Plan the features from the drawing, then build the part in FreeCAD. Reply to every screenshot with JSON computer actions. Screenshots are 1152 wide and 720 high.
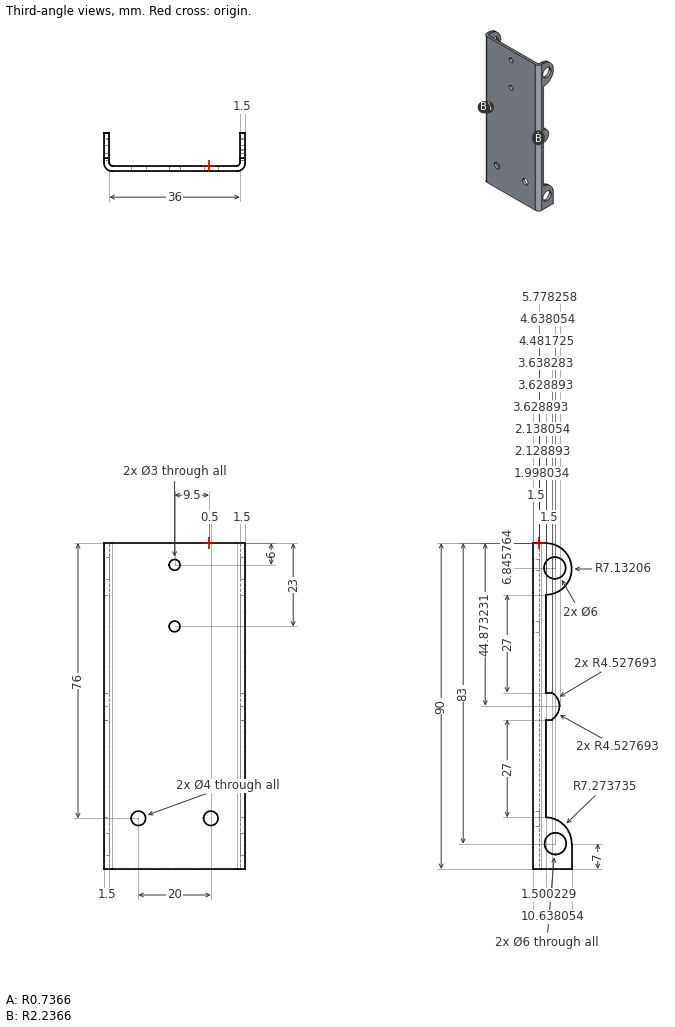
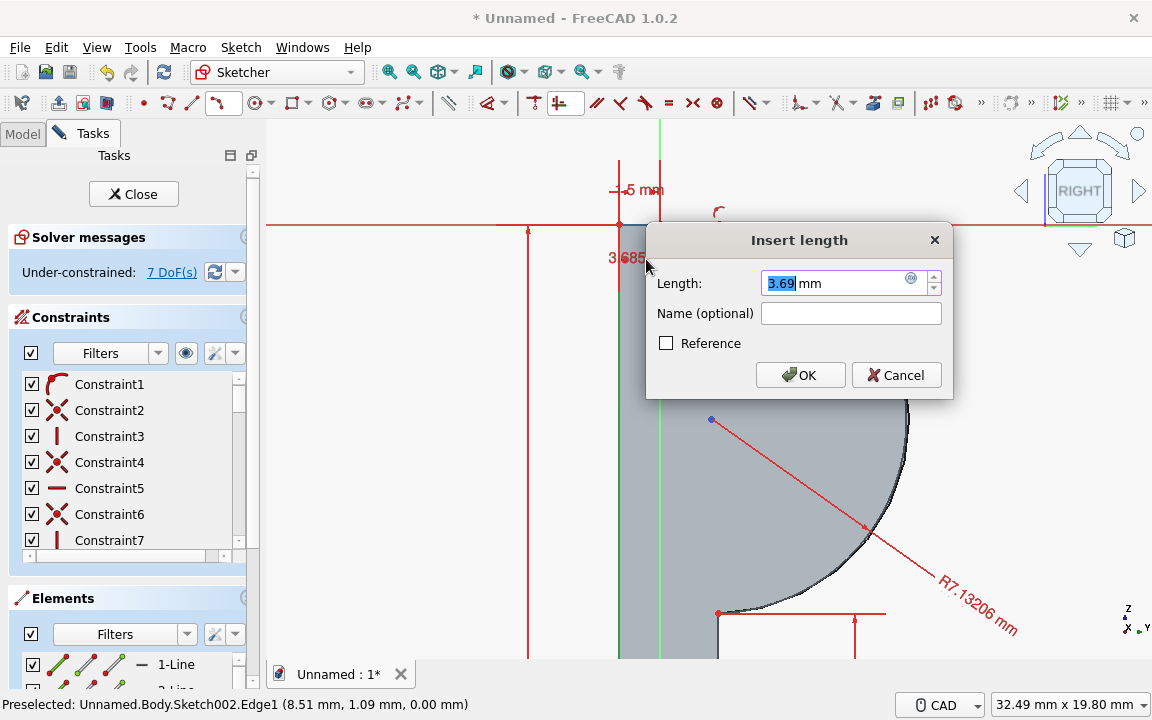
{"action": "type", "text": "3.628893"}
{"action": "key", "text": "Return"}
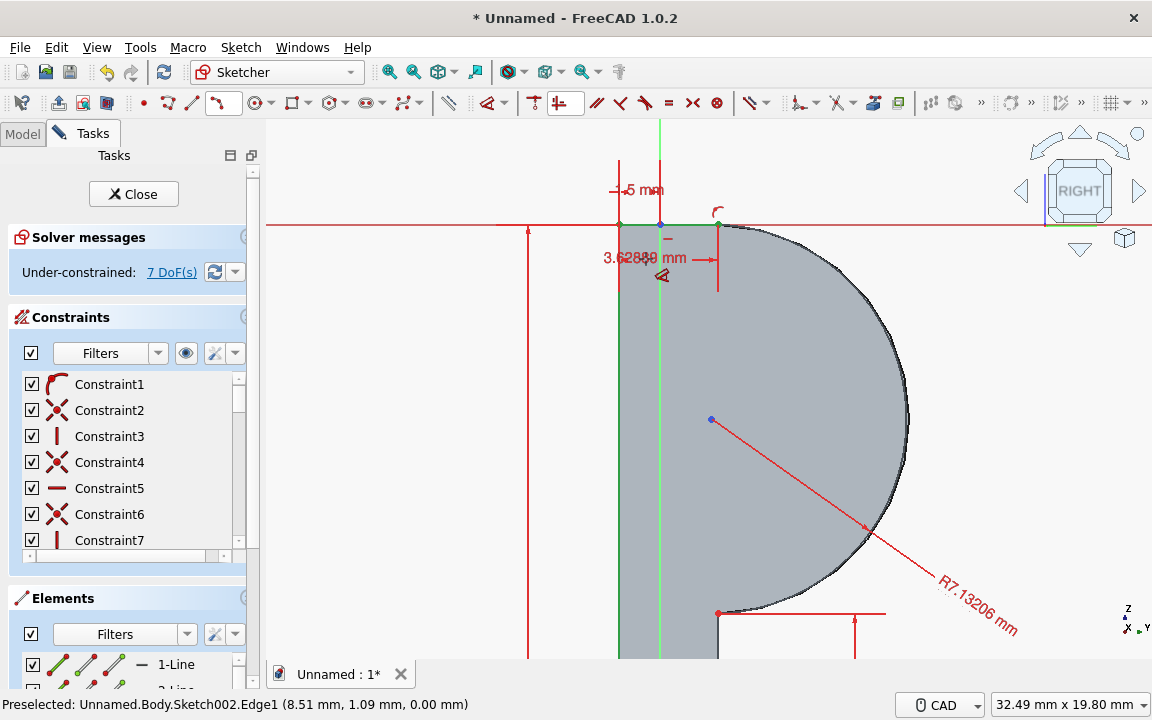
{"action": "scroll", "coordinate": [621, 223], "scroll_direction": "down", "scroll_amount": 10}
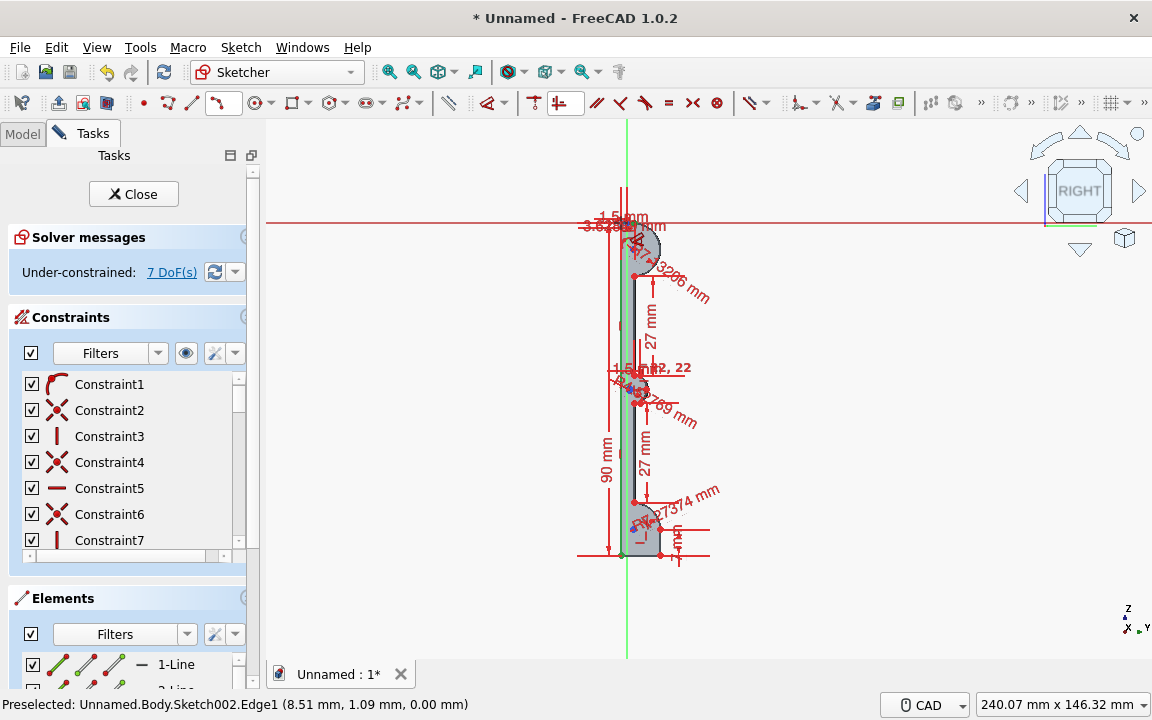
{"action": "scroll", "coordinate": [636, 403], "scroll_direction": "up", "scroll_amount": 11}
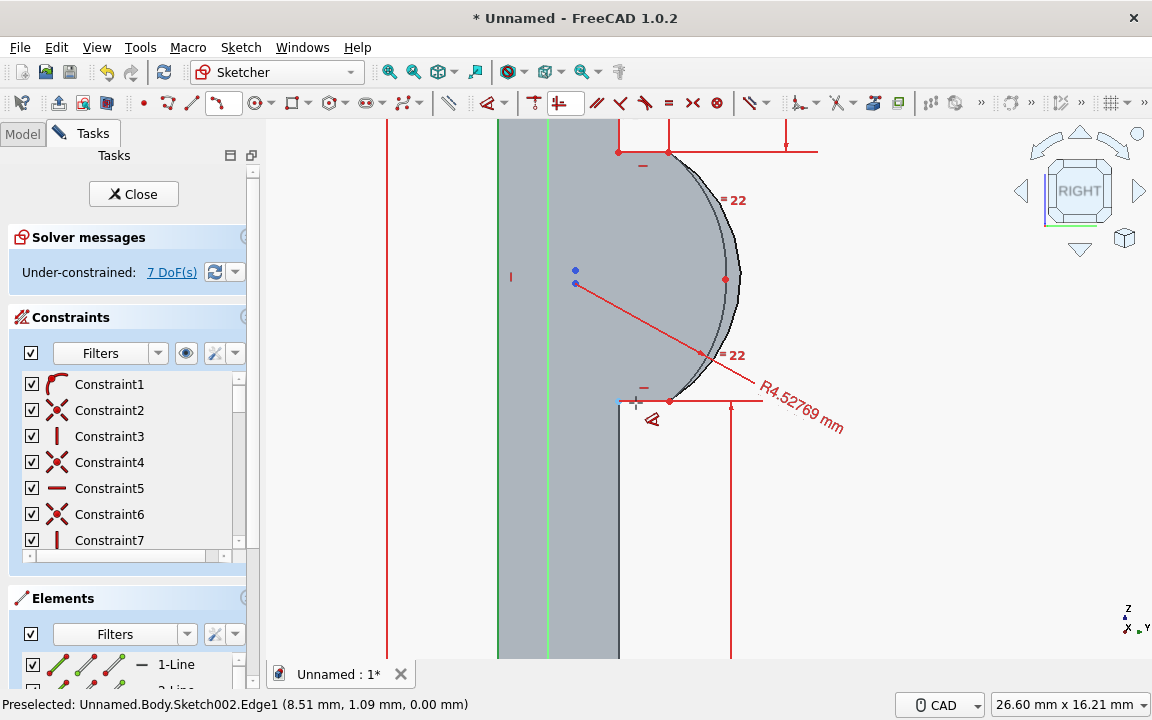
{"action": "left_click", "coordinate": [634, 401]}
{"action": "left_click", "coordinate": [644, 435]}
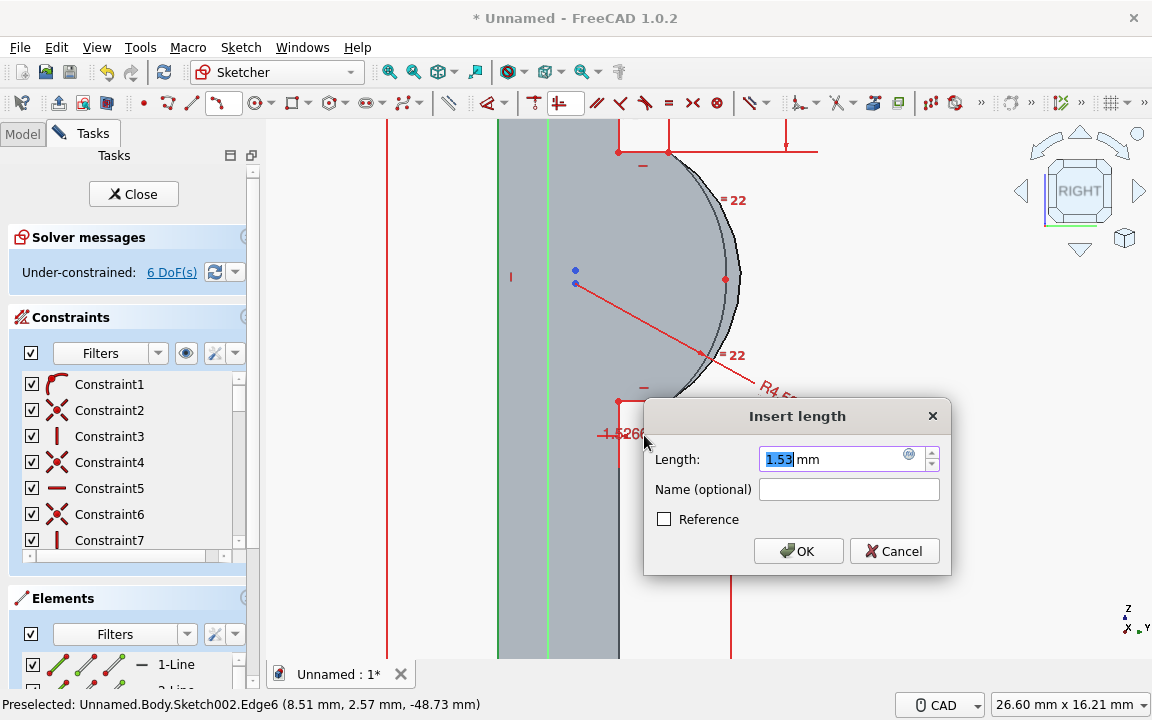
{"action": "type", "text": "1.500229"}
{"action": "key", "text": "Return"}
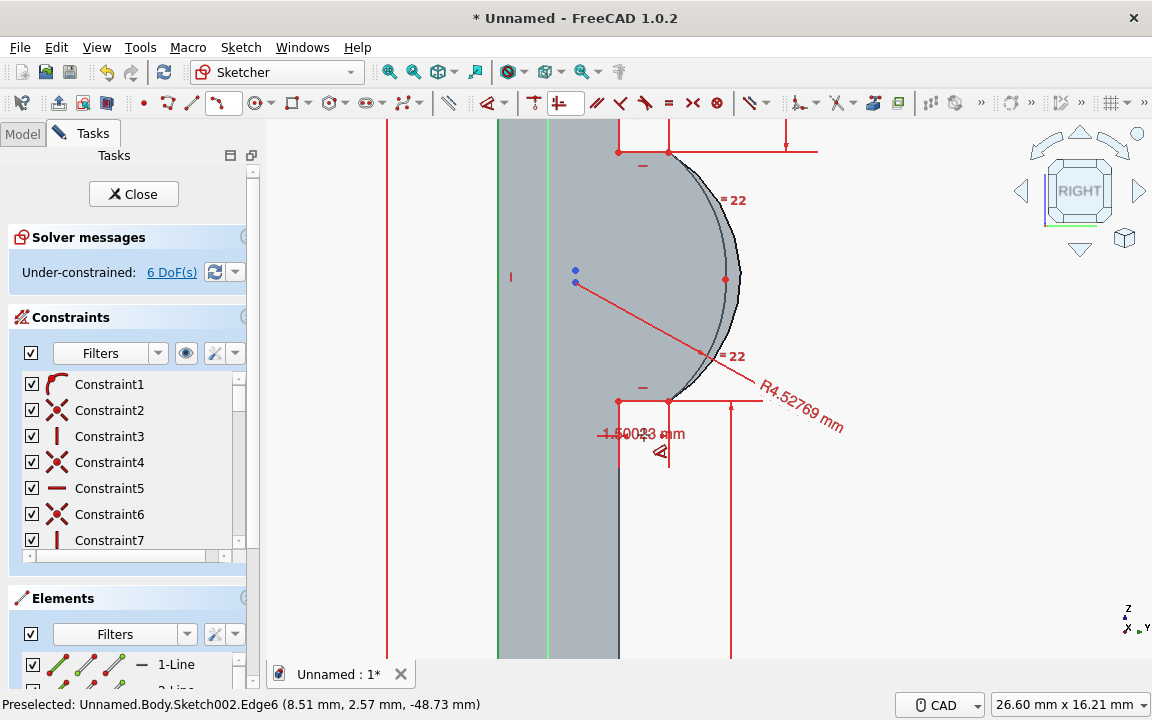
{"action": "scroll", "coordinate": [636, 403], "scroll_direction": "down", "scroll_amount": 11}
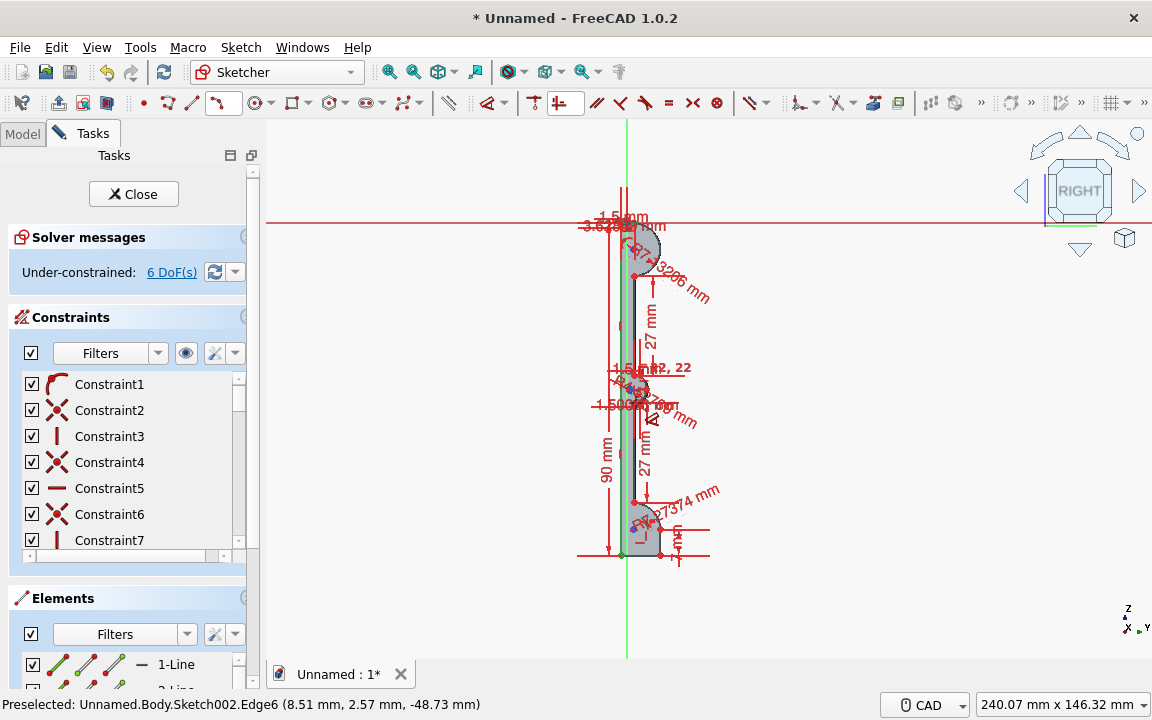
{"action": "scroll", "coordinate": [633, 556], "scroll_direction": "up", "scroll_amount": 4}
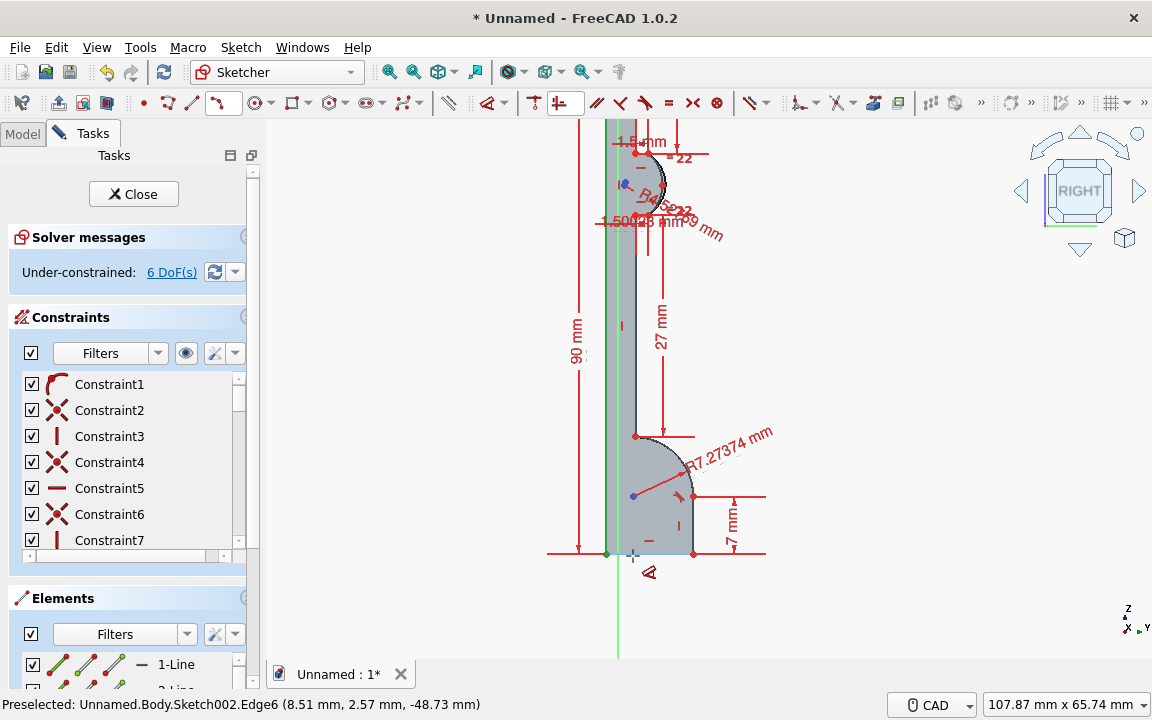
{"action": "left_click", "coordinate": [632, 554]}
{"action": "left_click", "coordinate": [650, 588]}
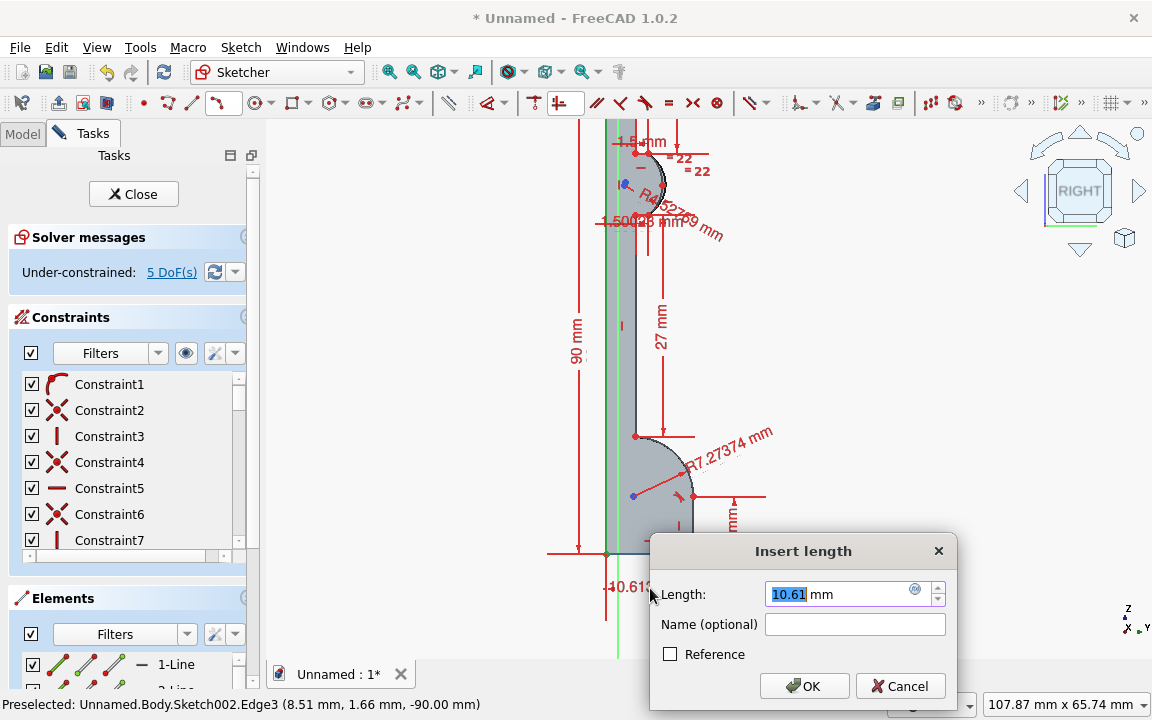
{"action": "type", "text": "10.638054"}
{"action": "key", "text": "Return"}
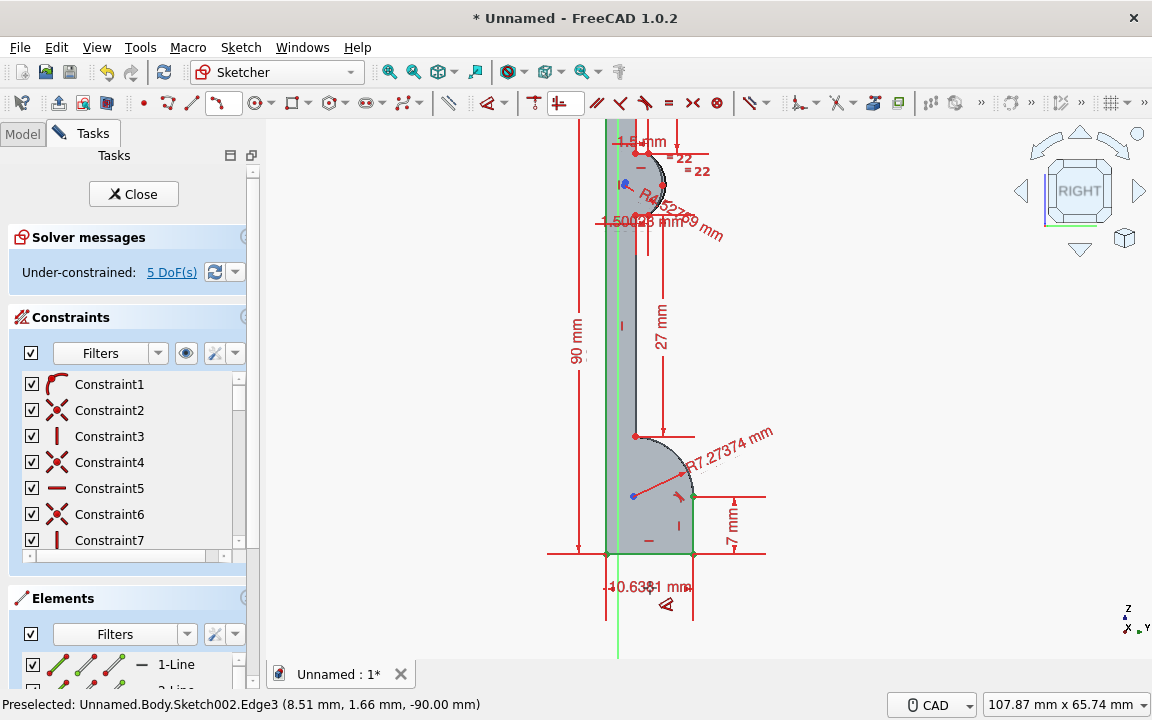
{"action": "scroll", "coordinate": [636, 437], "scroll_direction": "up", "scroll_amount": 5}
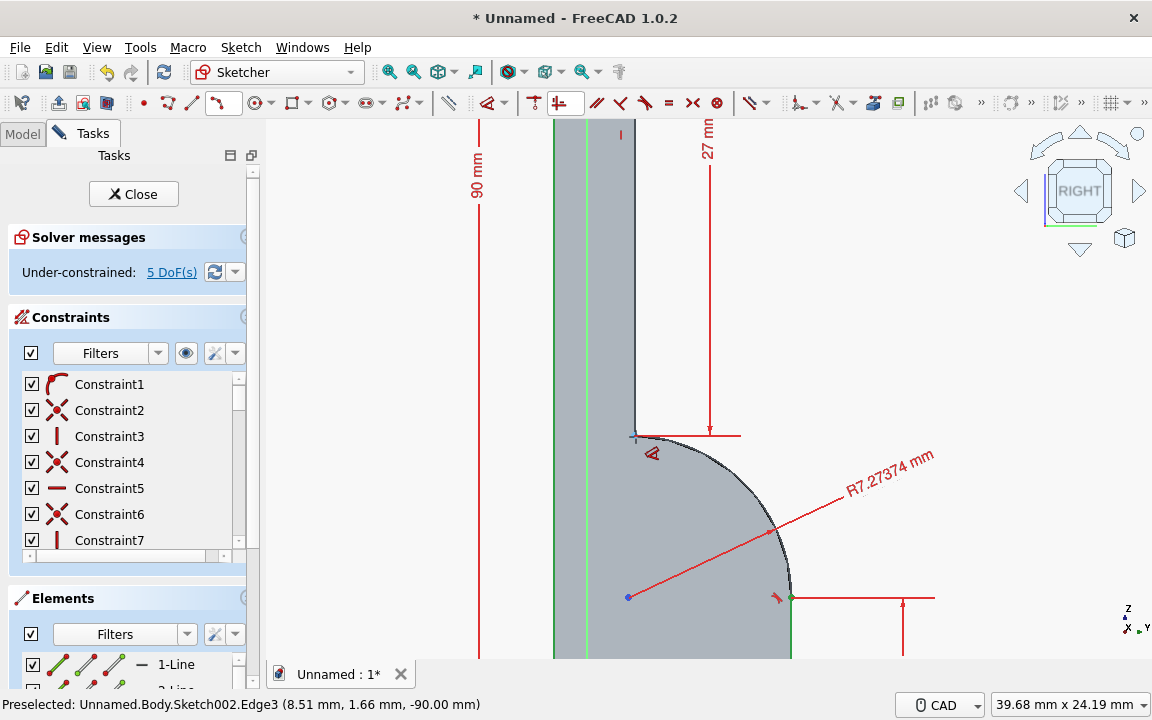
{"action": "left_click", "coordinate": [635, 436]}
{"action": "left_click", "coordinate": [611, 470]}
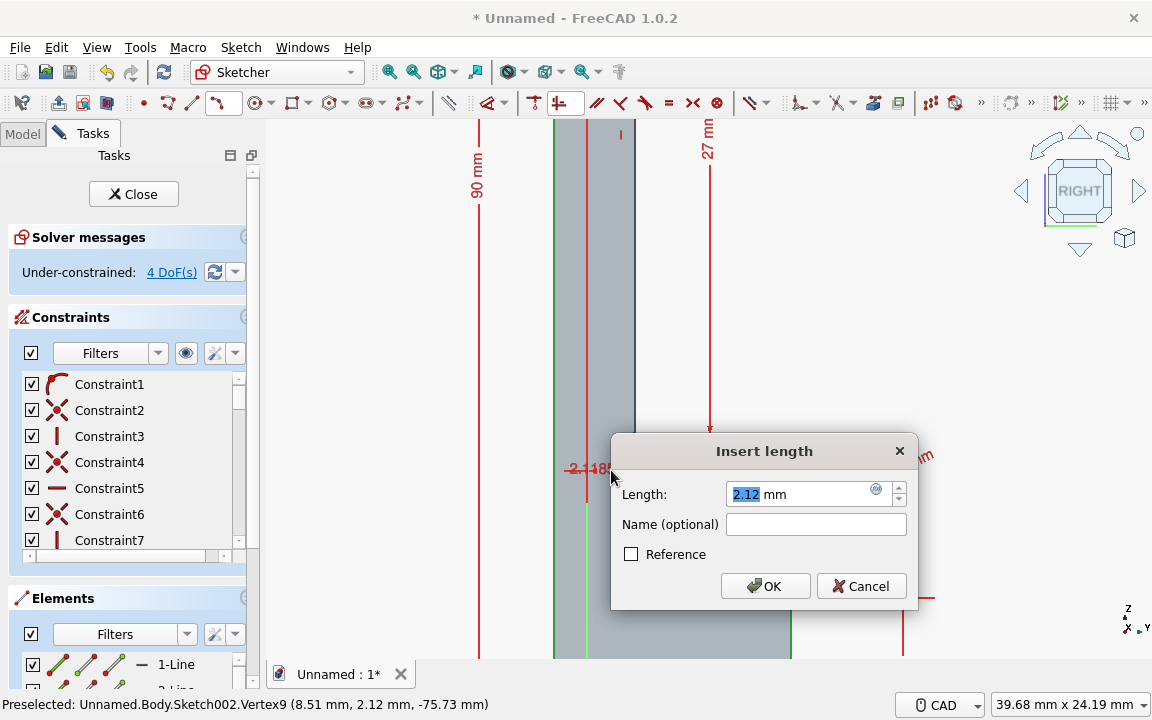
{"action": "type", "text": "2.138054"}
{"action": "key", "text": "Return"}